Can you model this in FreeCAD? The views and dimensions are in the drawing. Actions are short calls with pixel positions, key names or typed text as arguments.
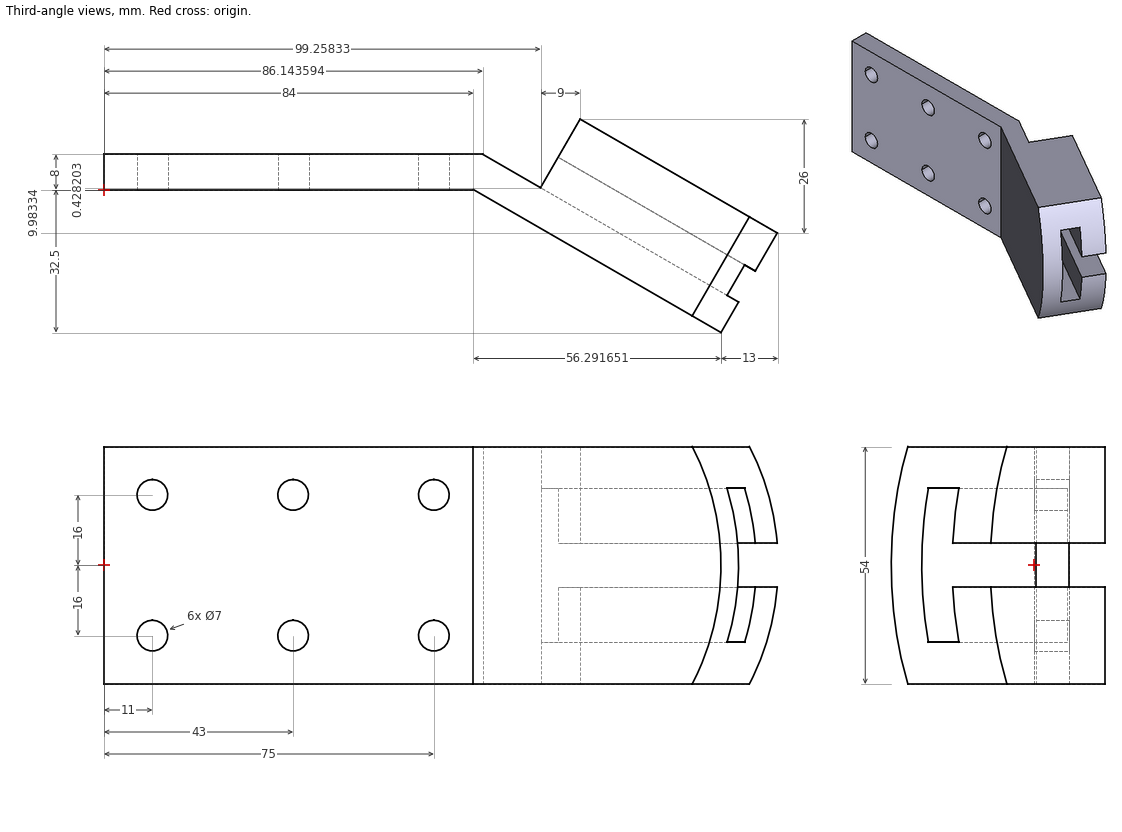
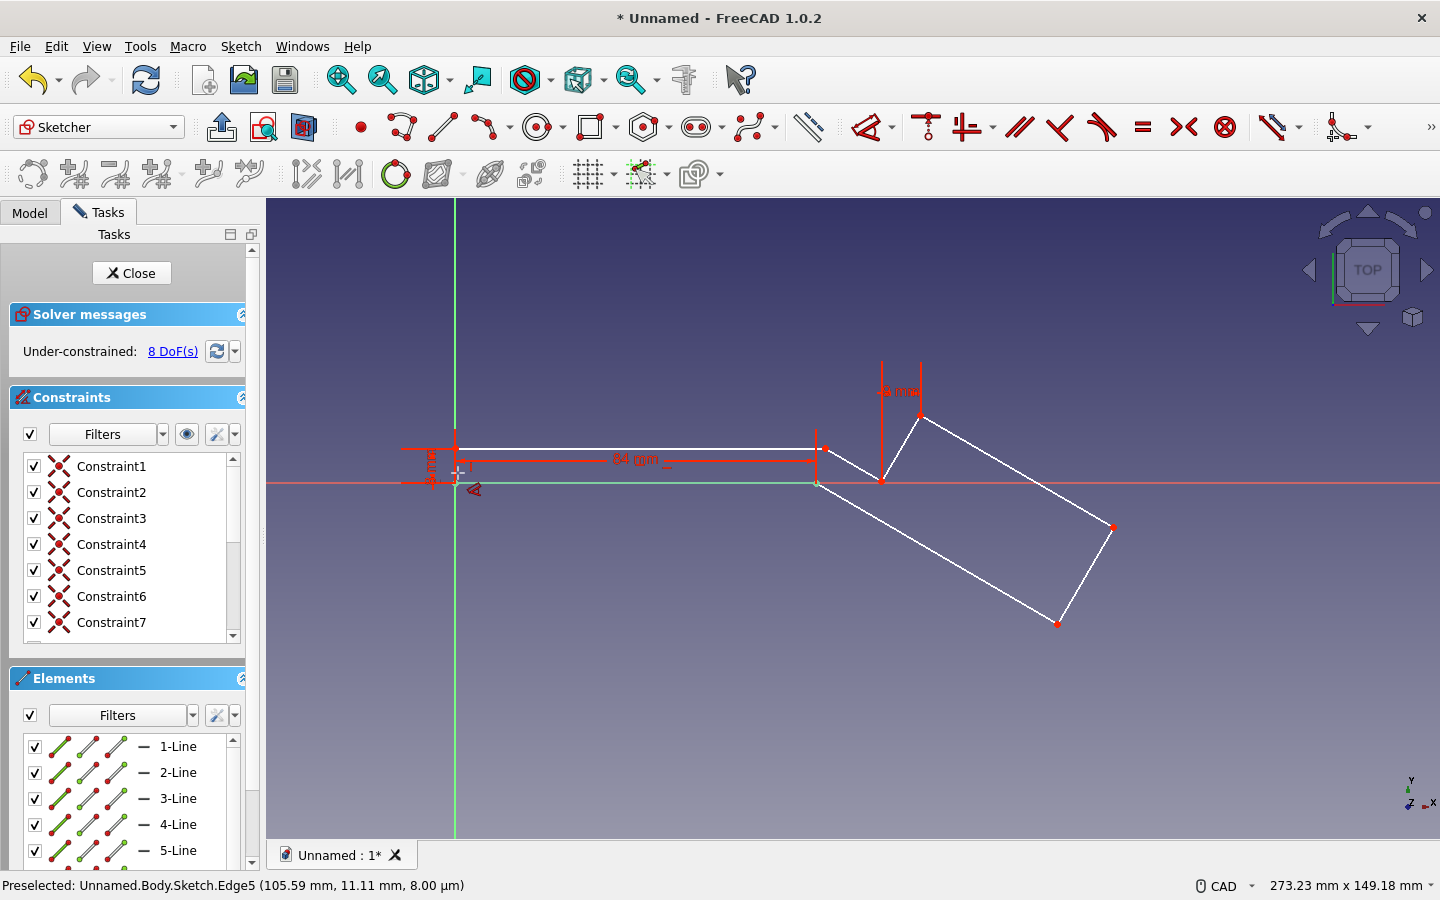
click(1075, 595)
click(1086, 658)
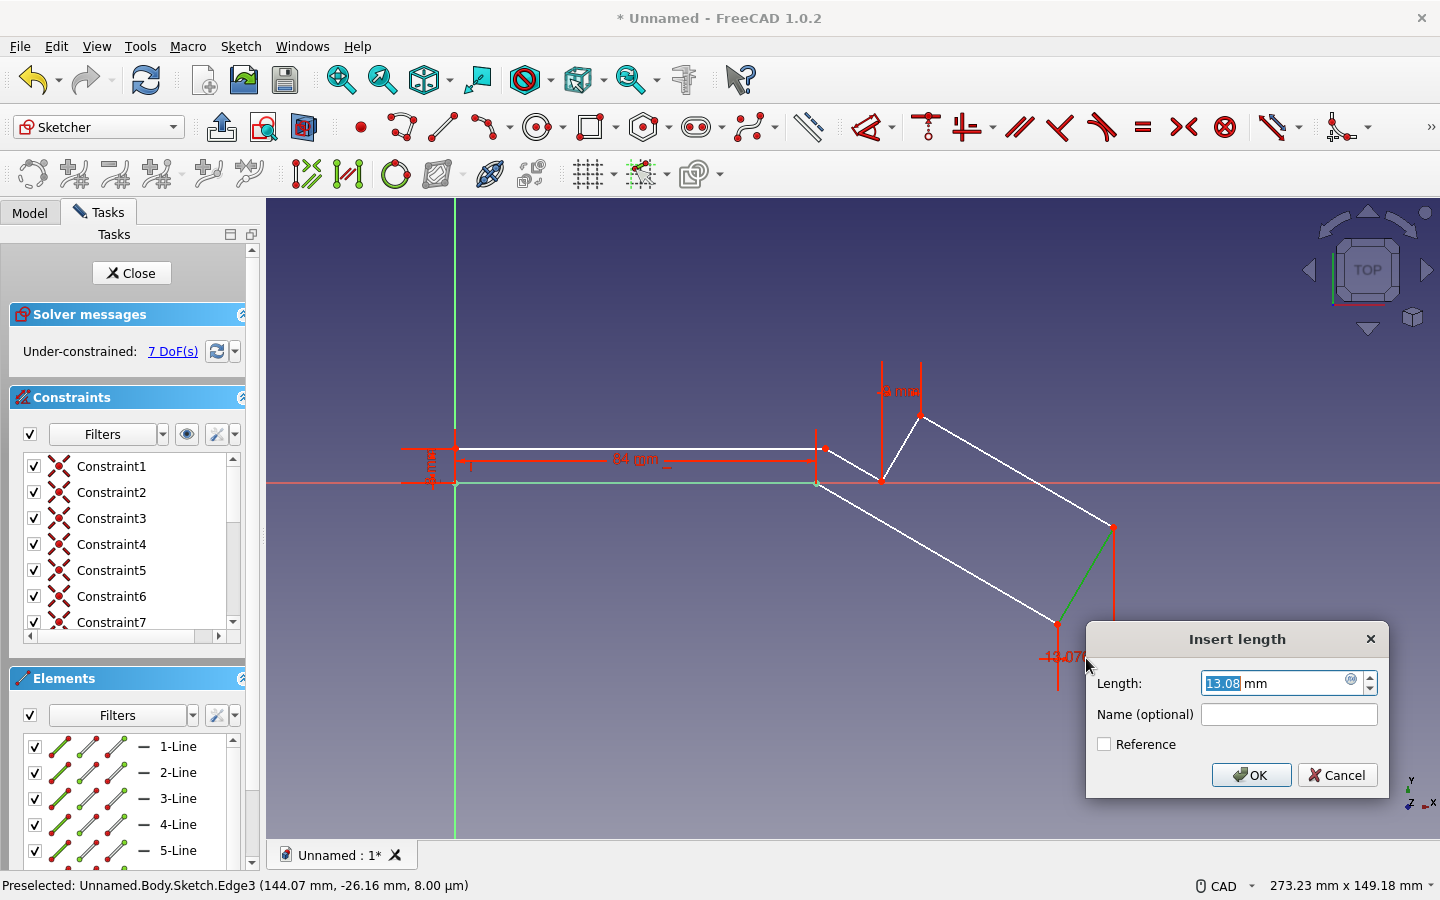
text(13)
key(Return)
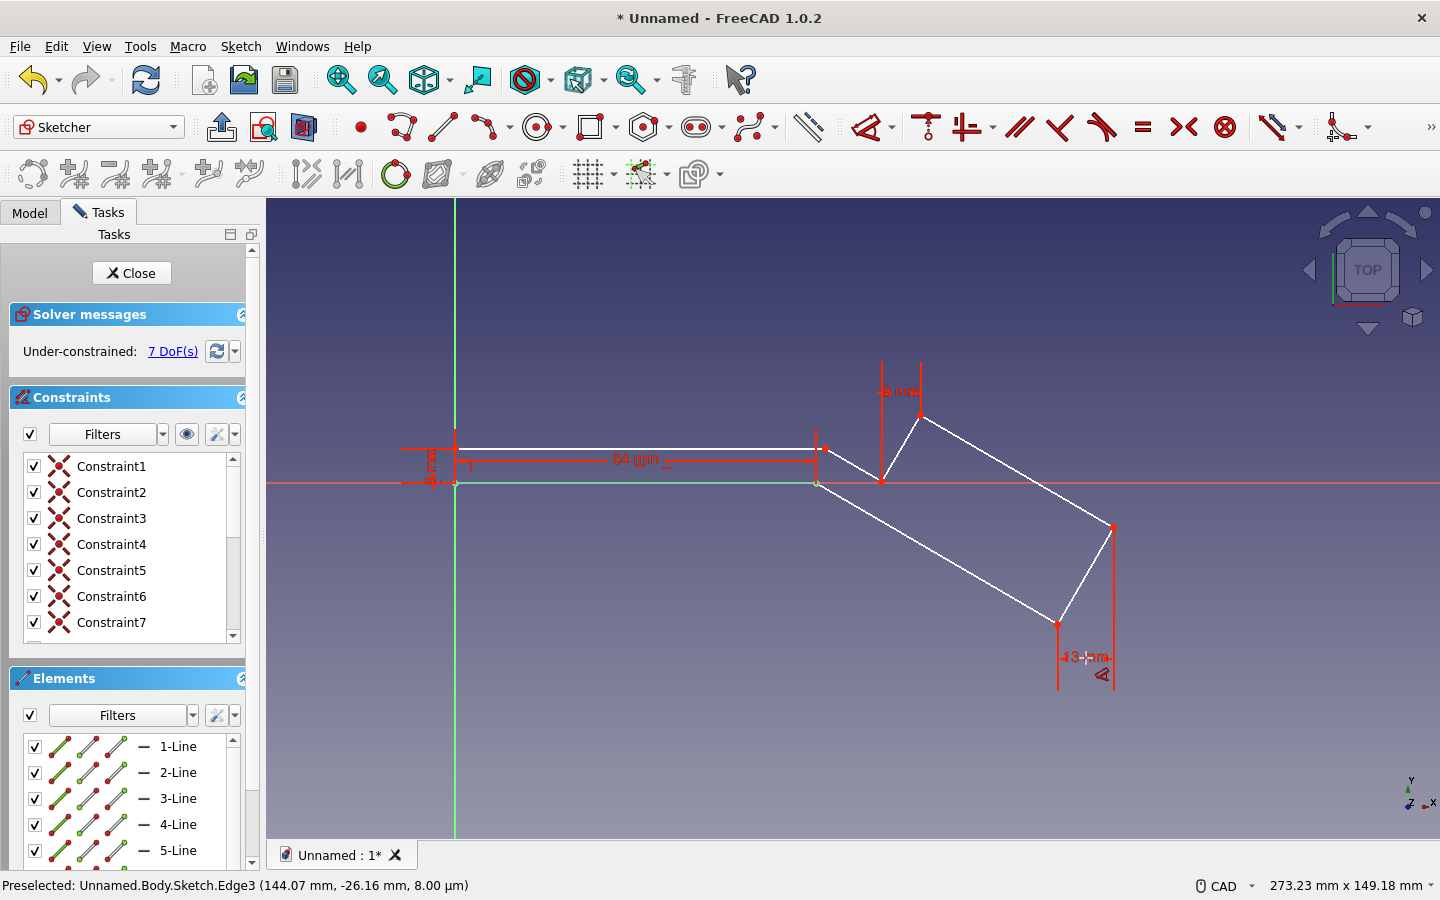
scroll(1056, 494, up, 2)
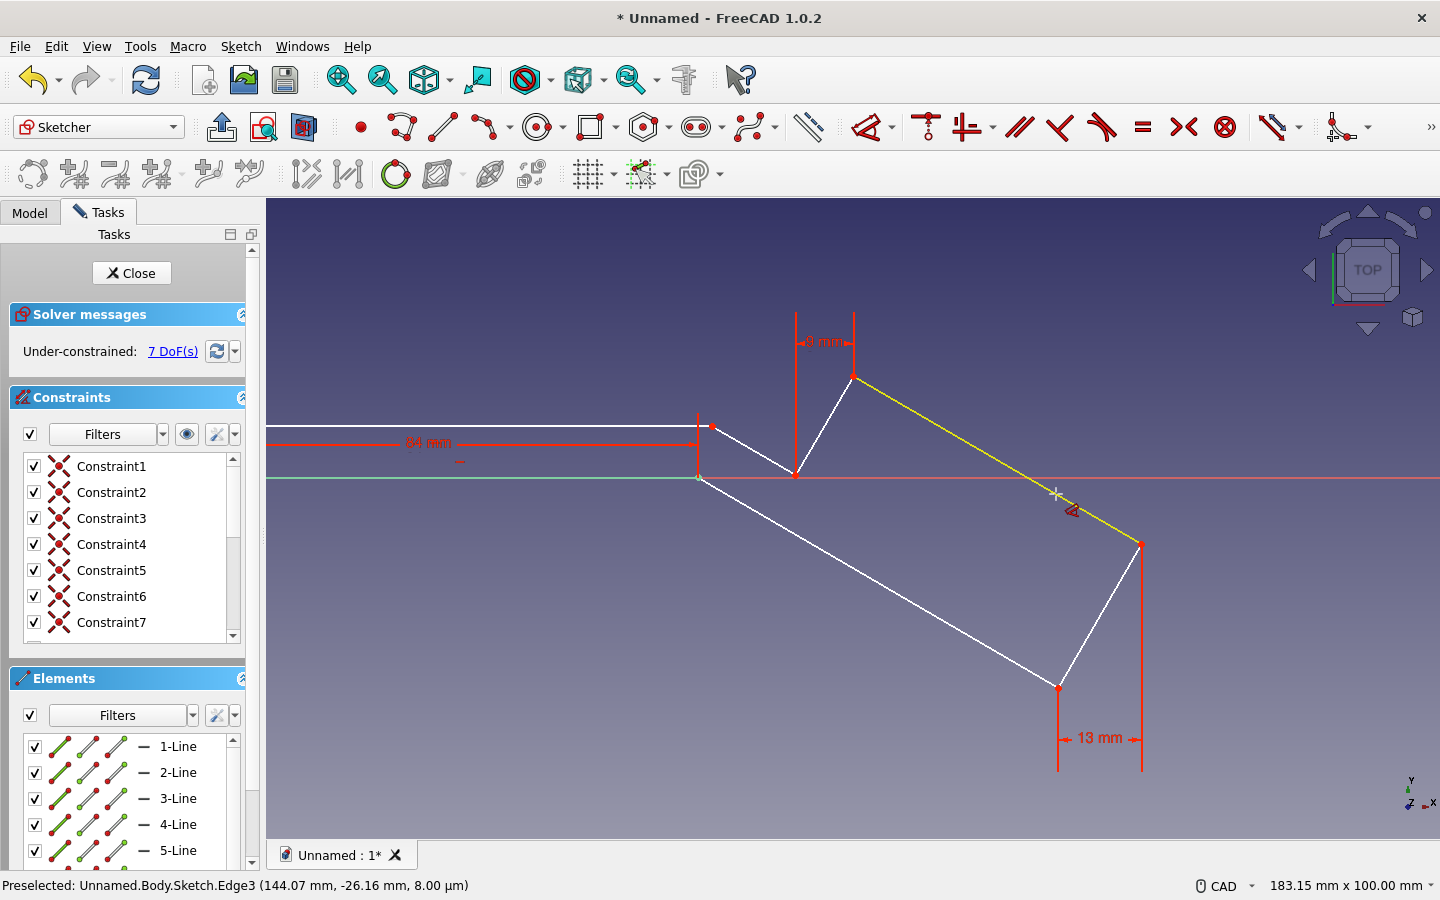
click(1055, 494)
click(1176, 460)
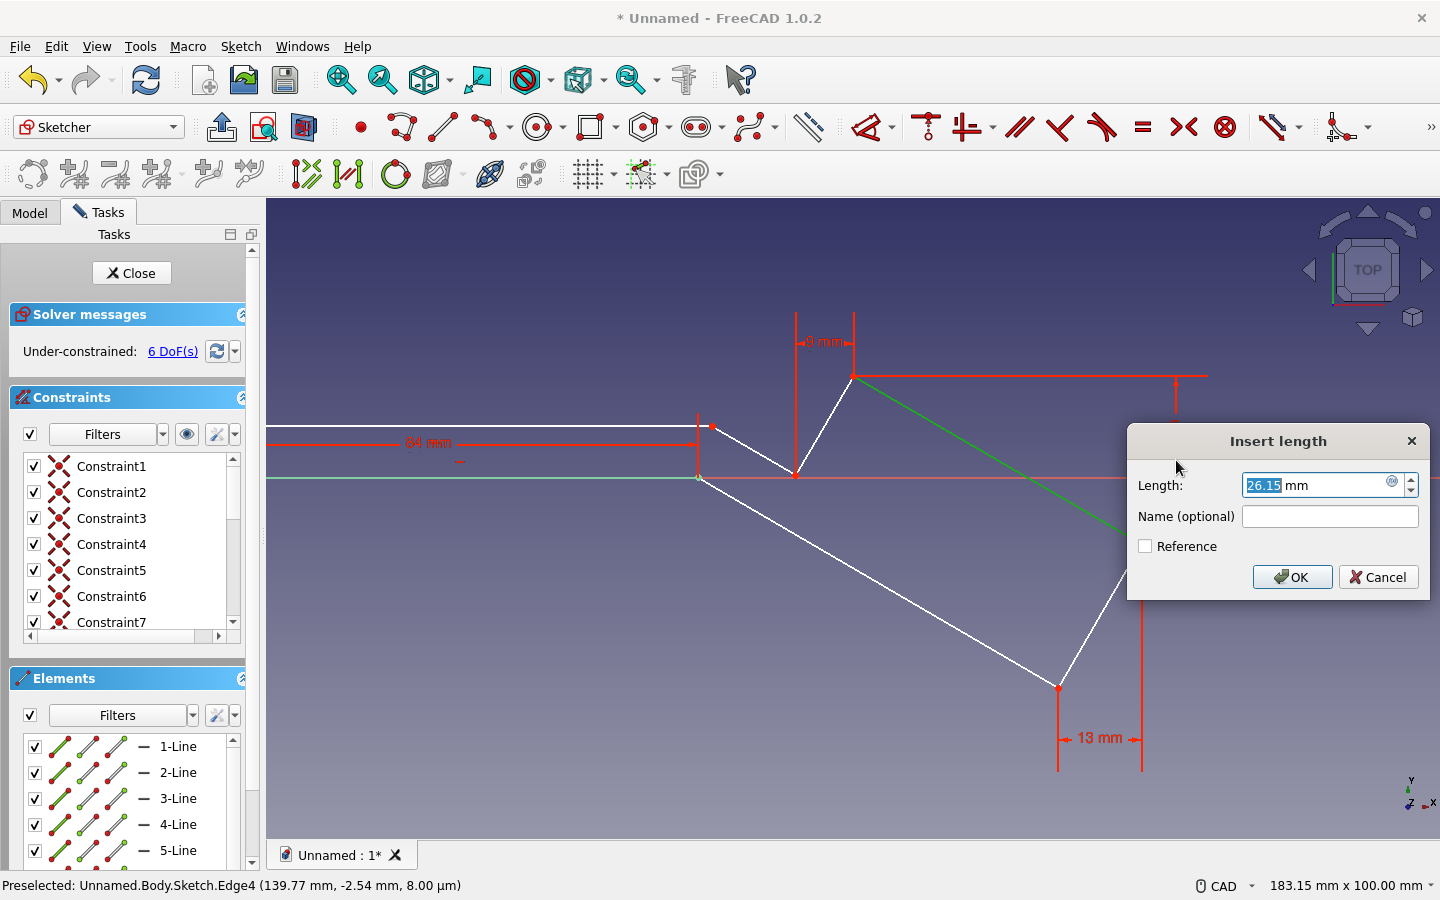
text(26)
key(Return)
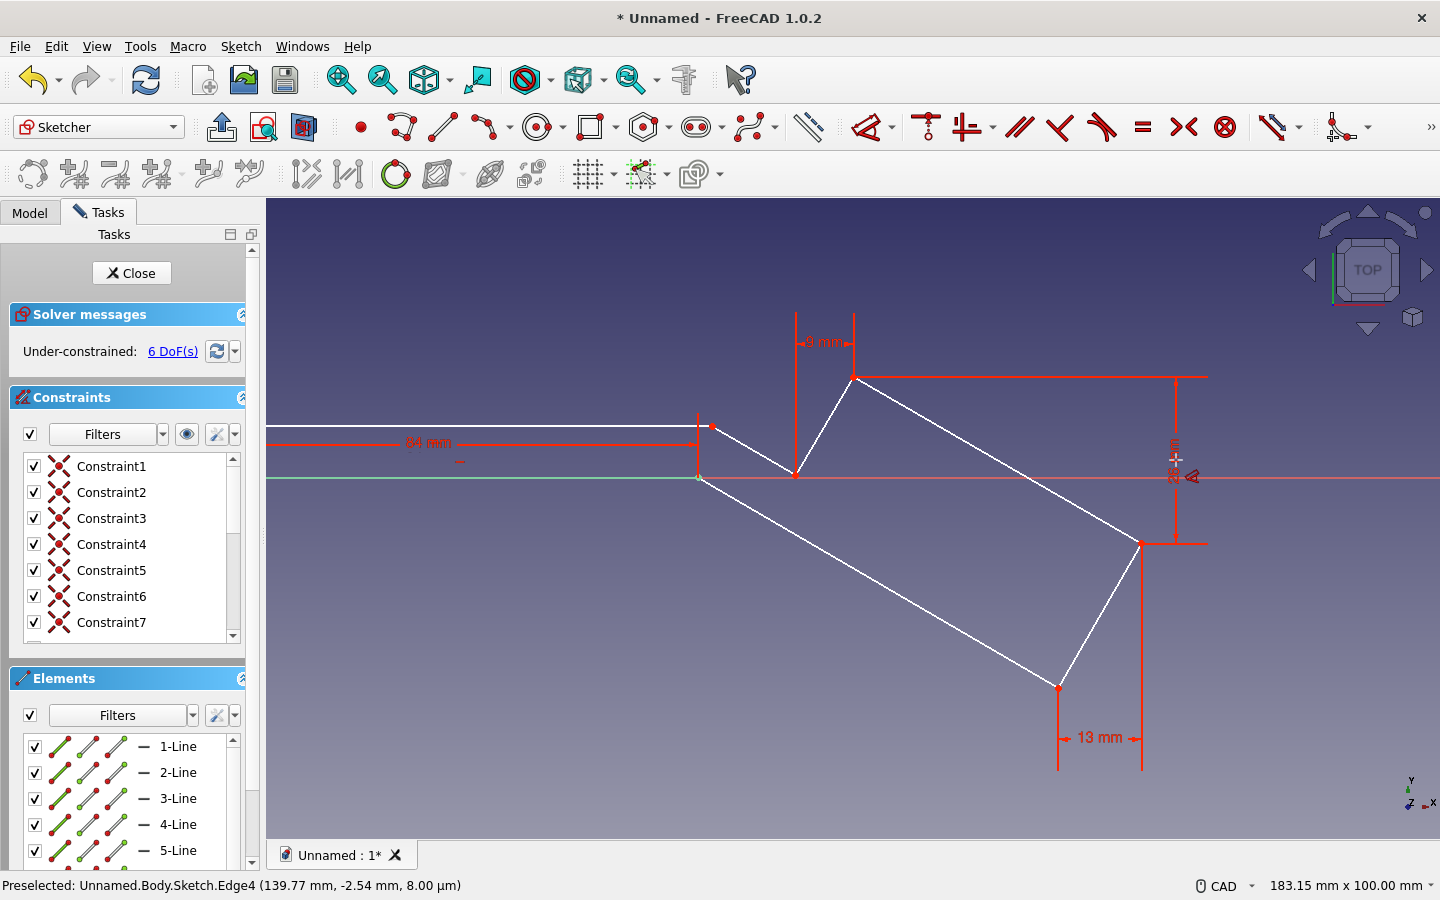
click(1058, 688)
click(1092, 583)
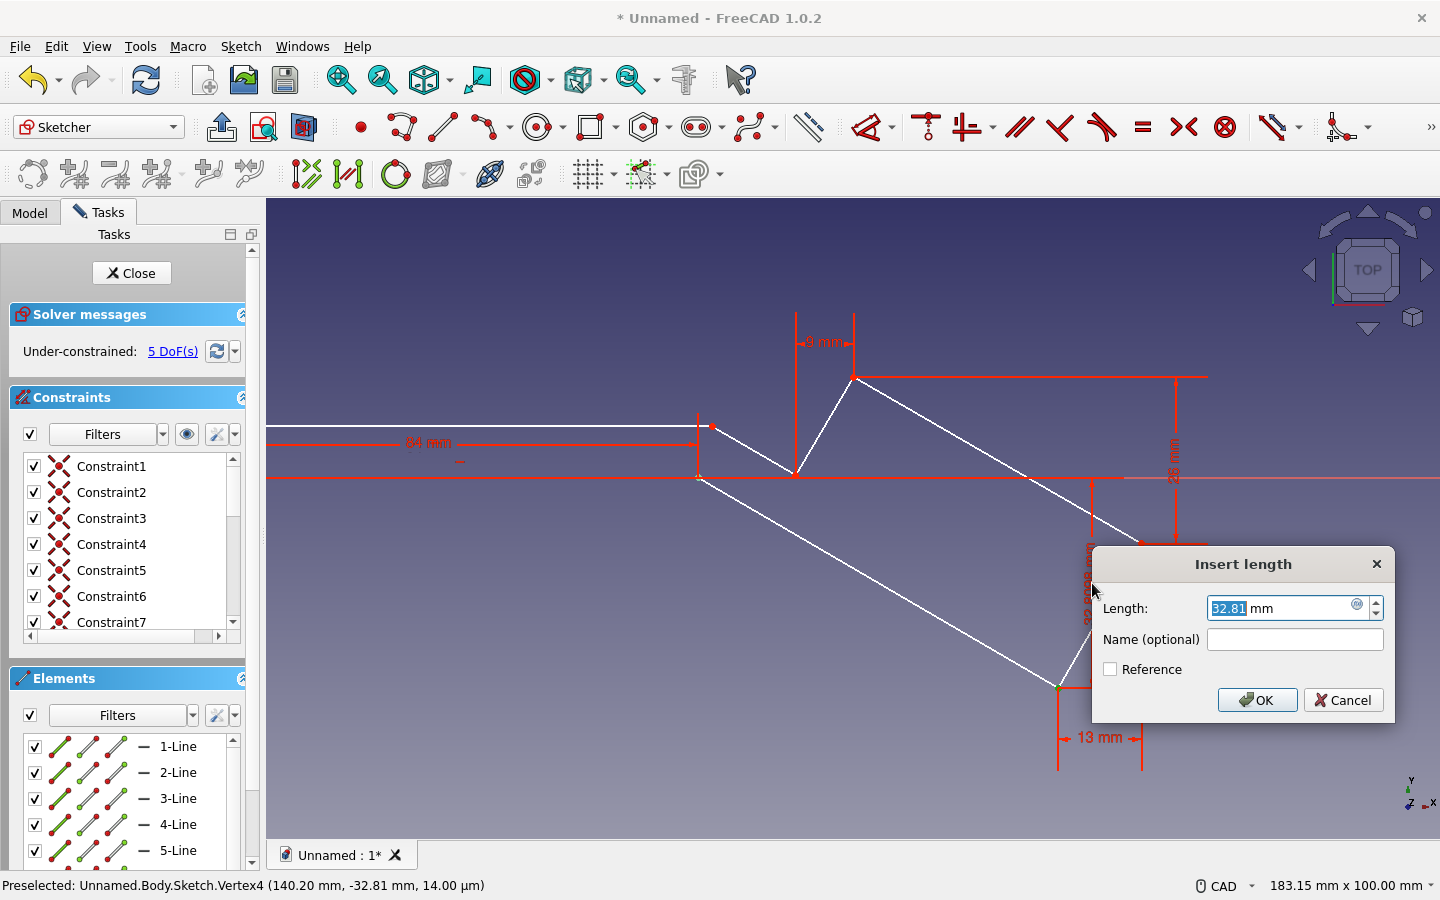
text(32.5)
key(Return)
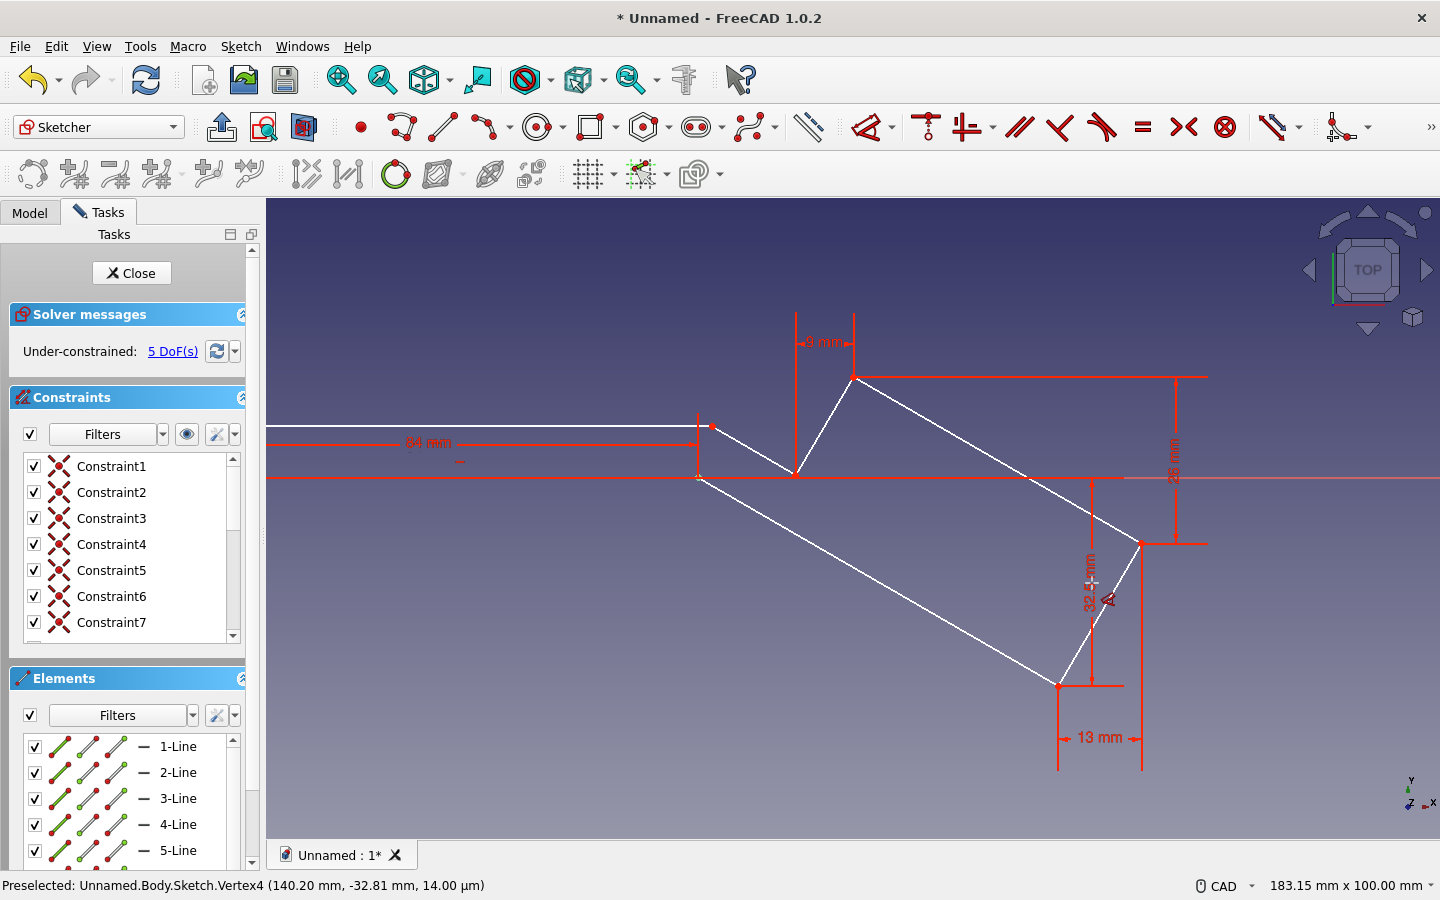
click(1142, 544)
click(1176, 511)